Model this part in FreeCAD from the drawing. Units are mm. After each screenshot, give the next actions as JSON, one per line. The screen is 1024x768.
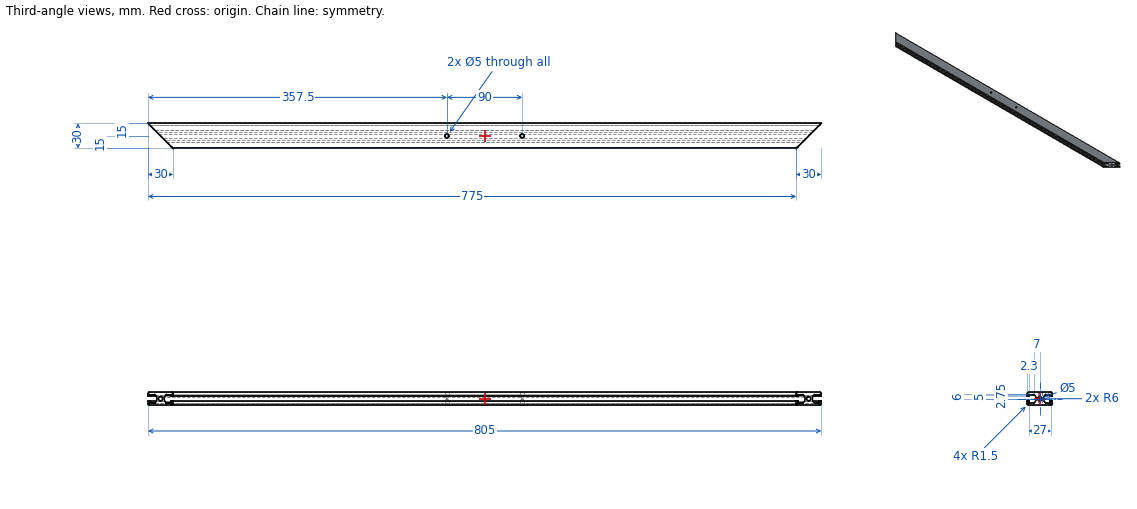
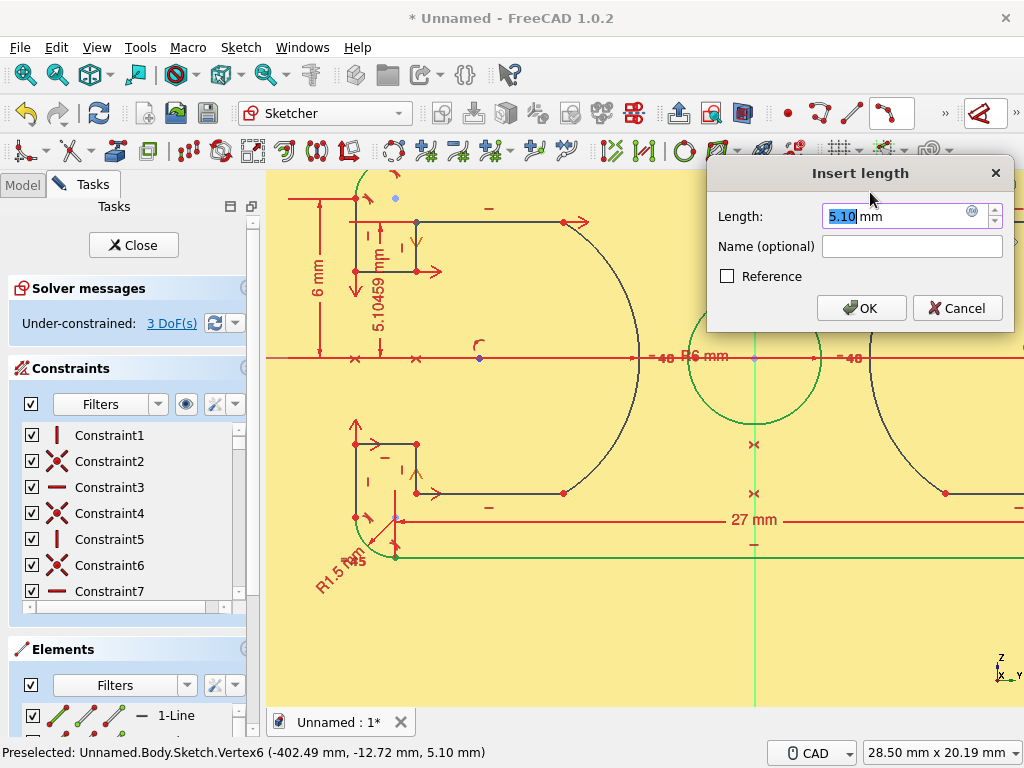
{"action": "type", "text": "5"}
{"action": "key", "text": "Return"}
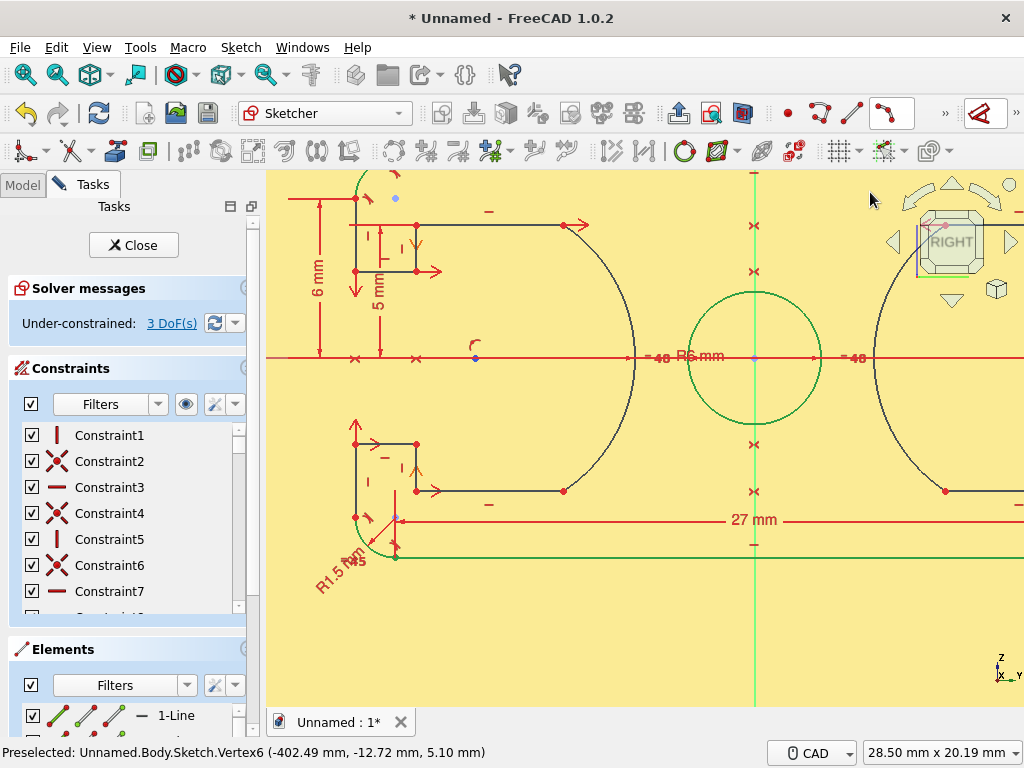
{"action": "left_click", "coordinate": [564, 225]}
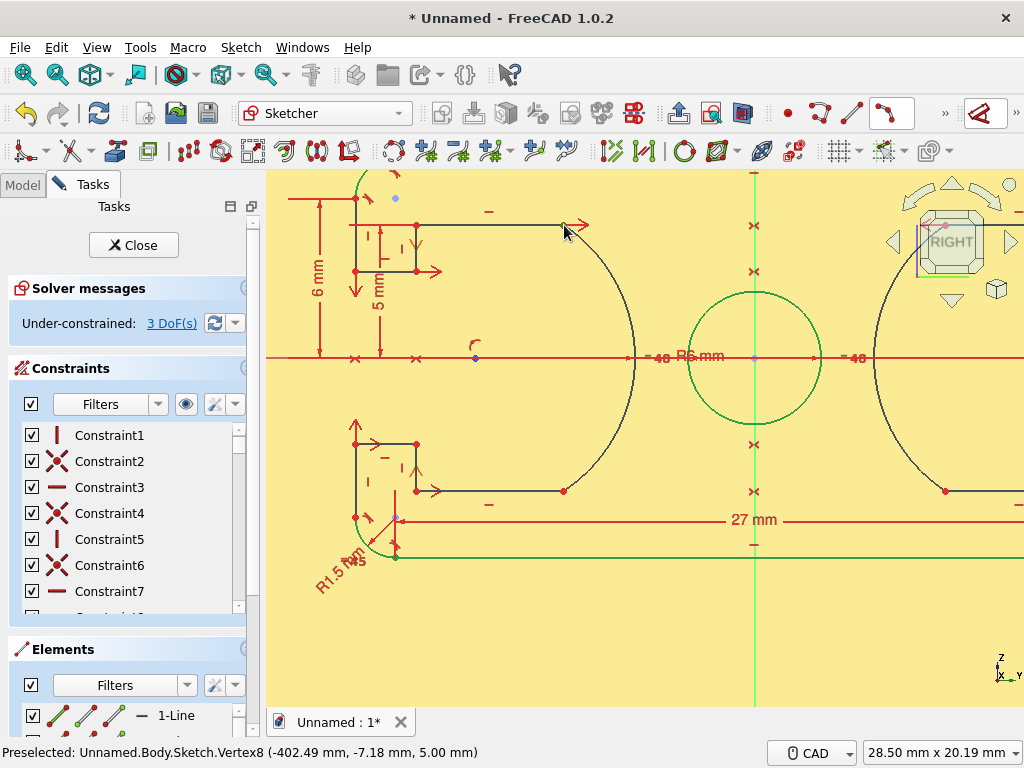
{"action": "left_click", "coordinate": [1002, 114]}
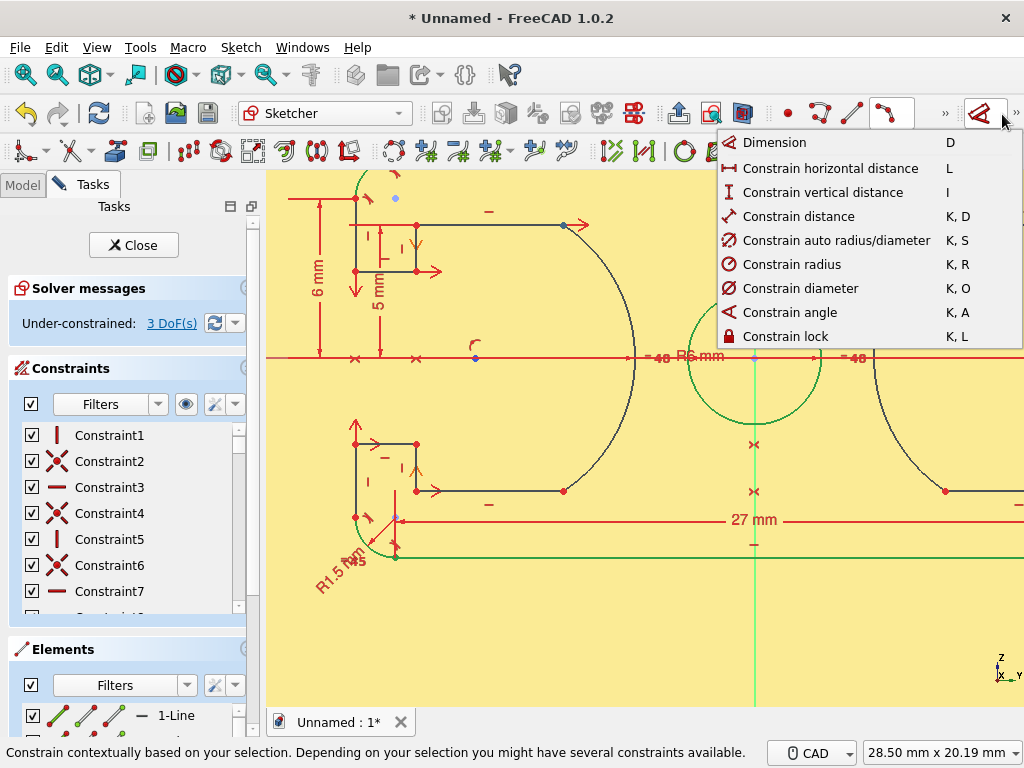
{"action": "left_click", "coordinate": [870, 168]}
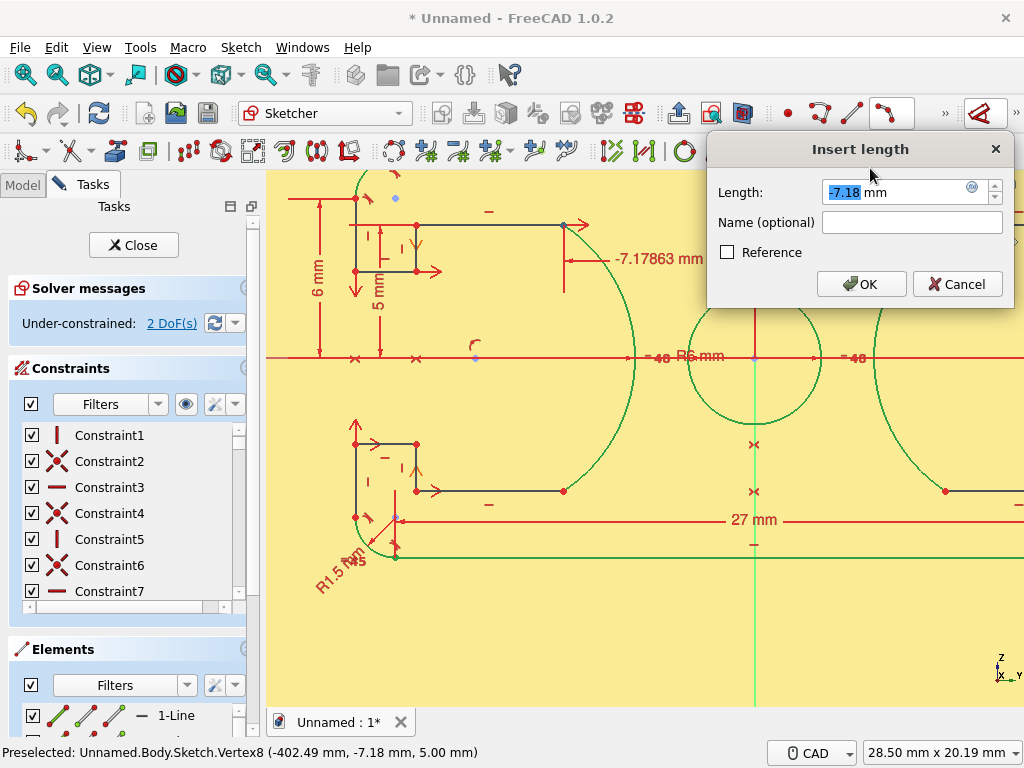
{"action": "type", "text": "-7"}
{"action": "key", "text": "Return"}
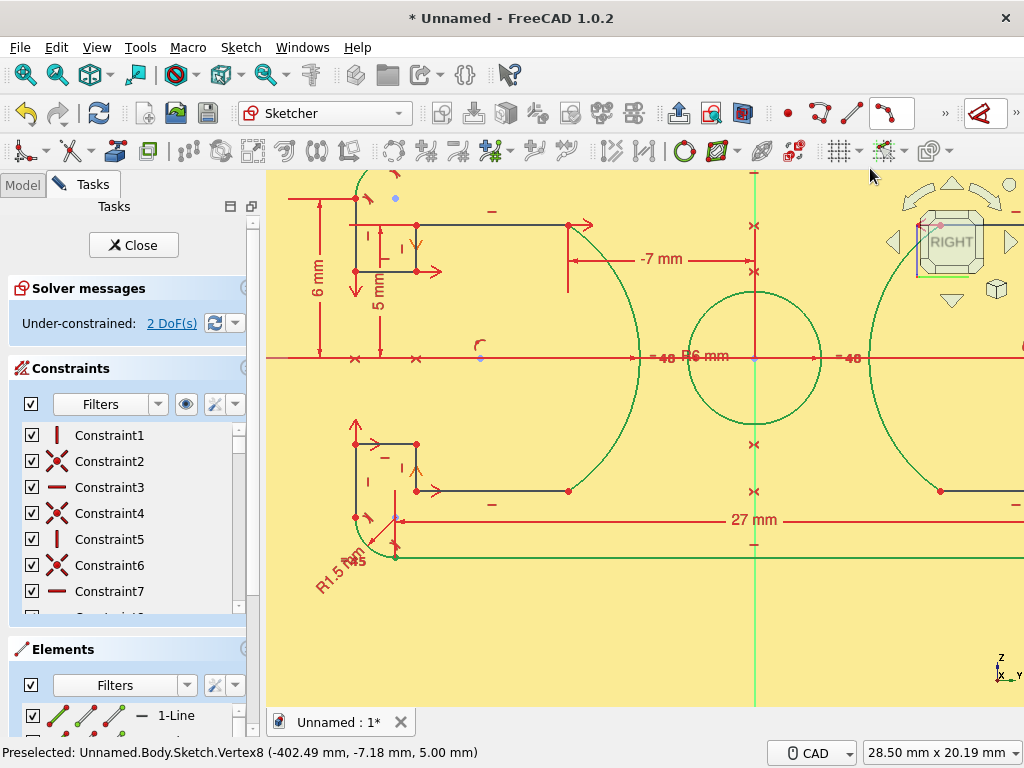
{"action": "left_click", "coordinate": [374, 272]}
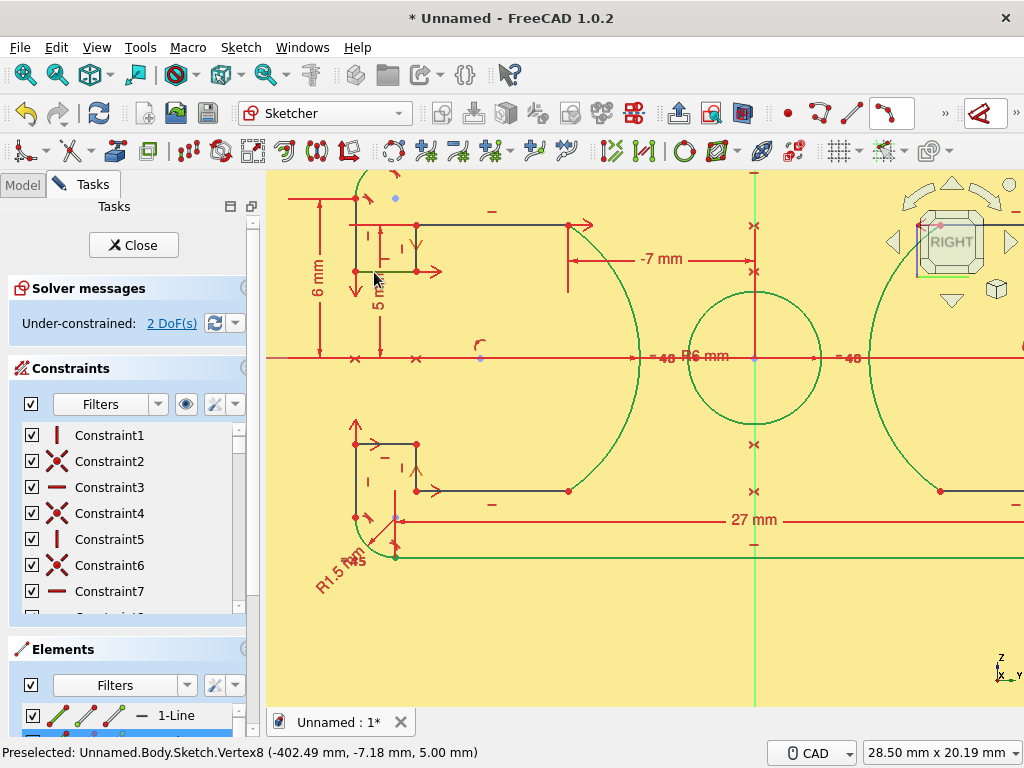
{"action": "left_click", "coordinate": [1002, 114]}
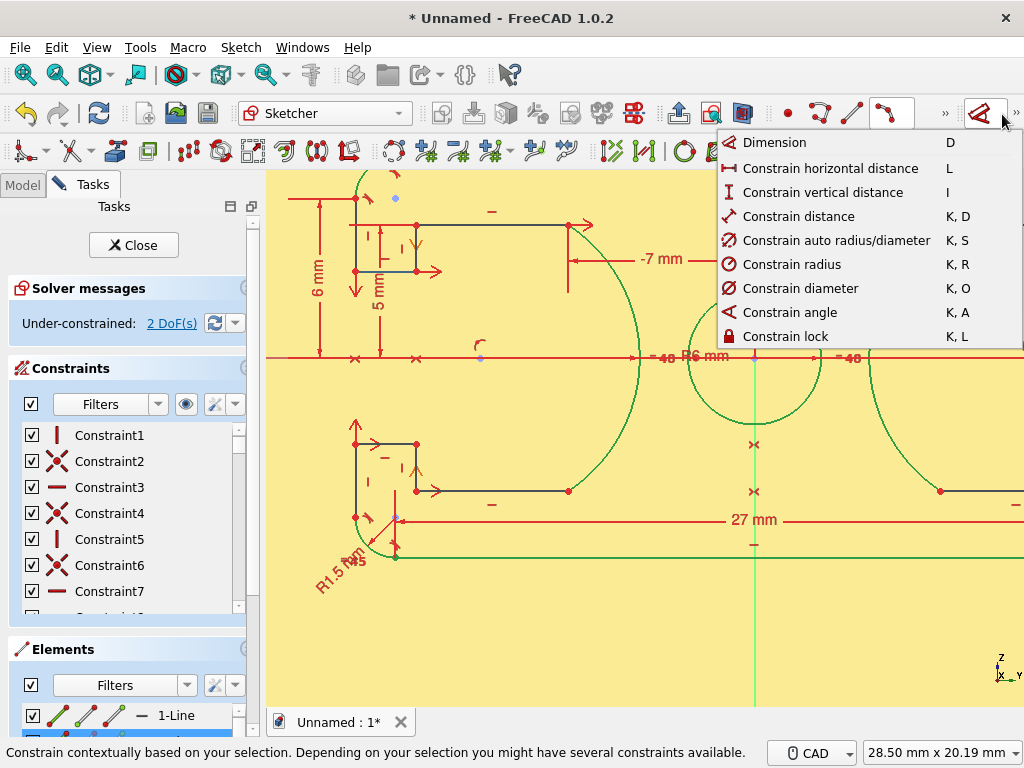
{"action": "left_click", "coordinate": [870, 168]}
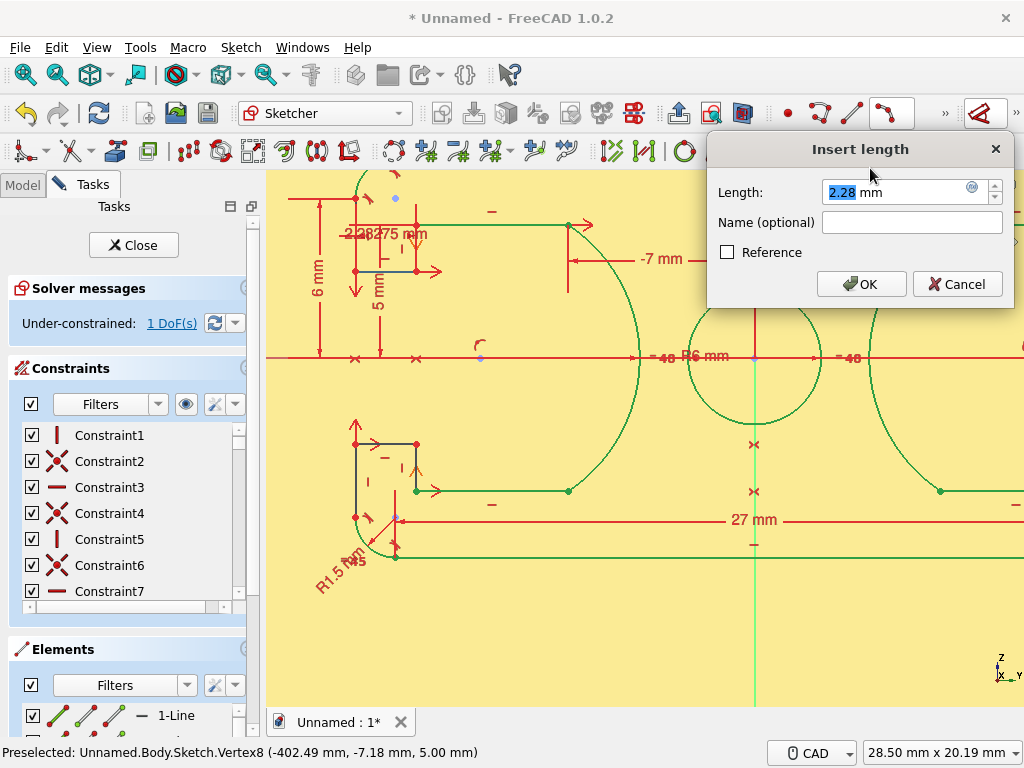
{"action": "type", "text": "2.3"}
{"action": "key", "text": "Return"}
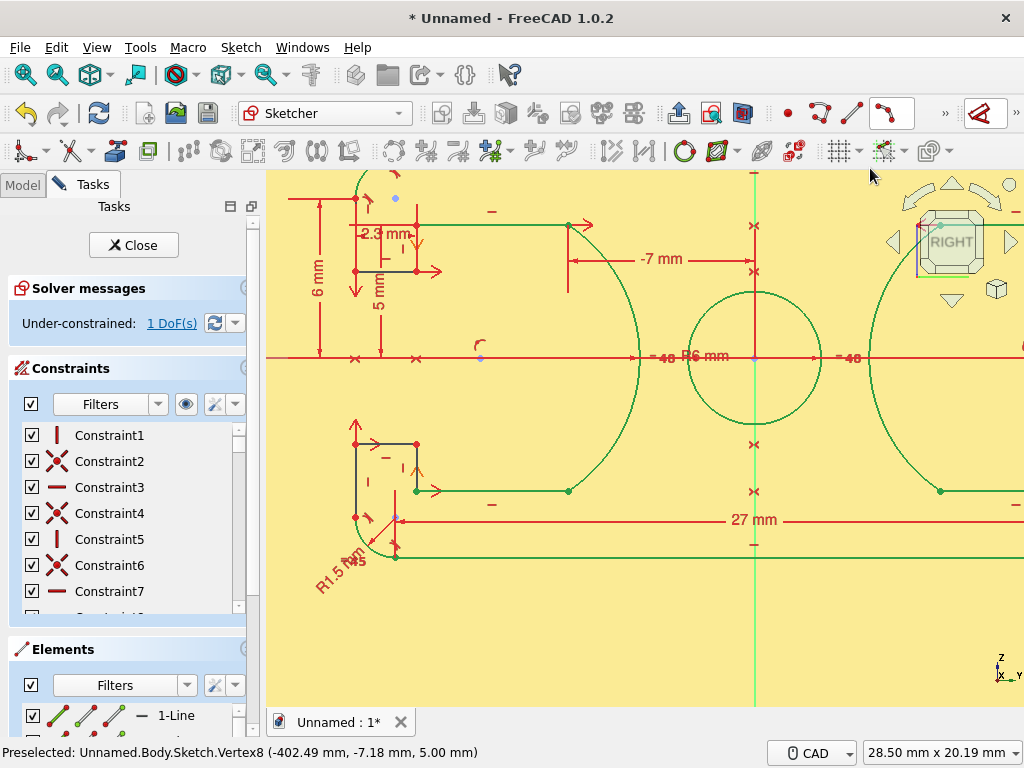
{"action": "left_click", "coordinate": [356, 220]}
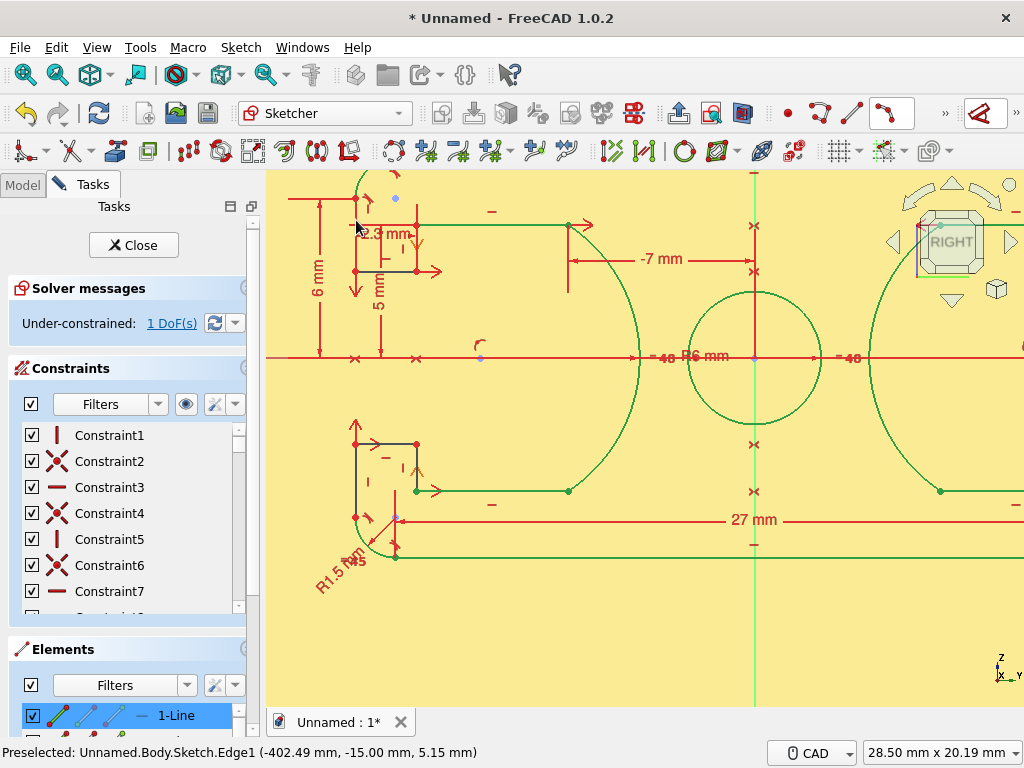
{"action": "key", "text": "i"}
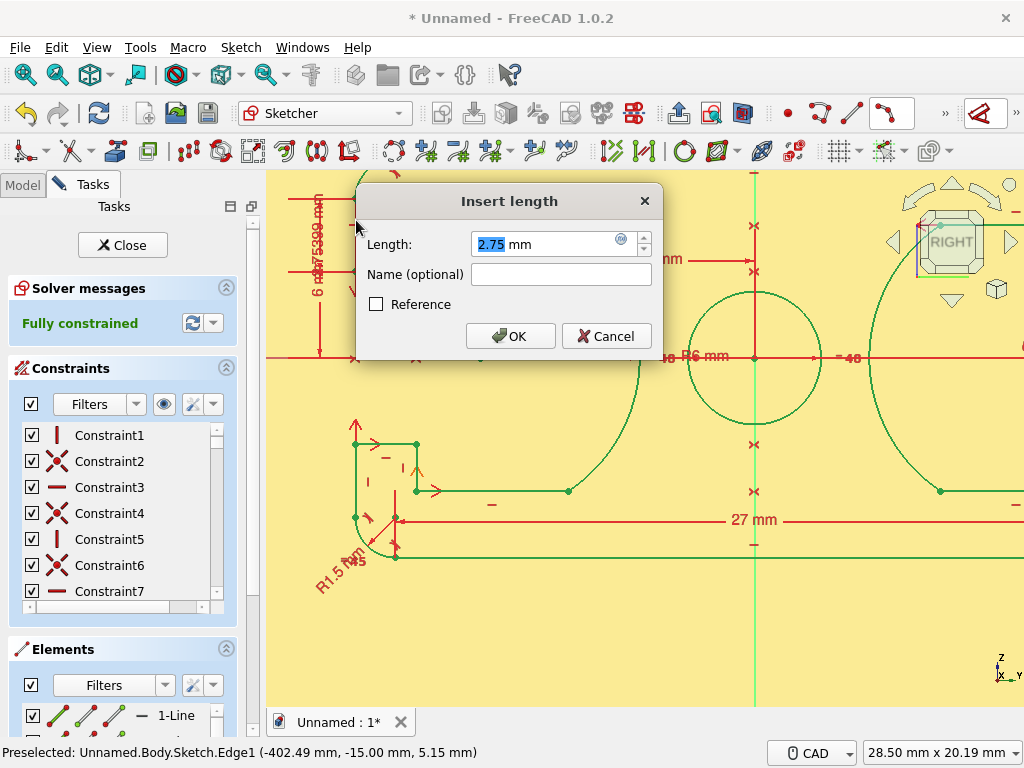
{"action": "type", "text": "2.75"}
{"action": "key", "text": "Return"}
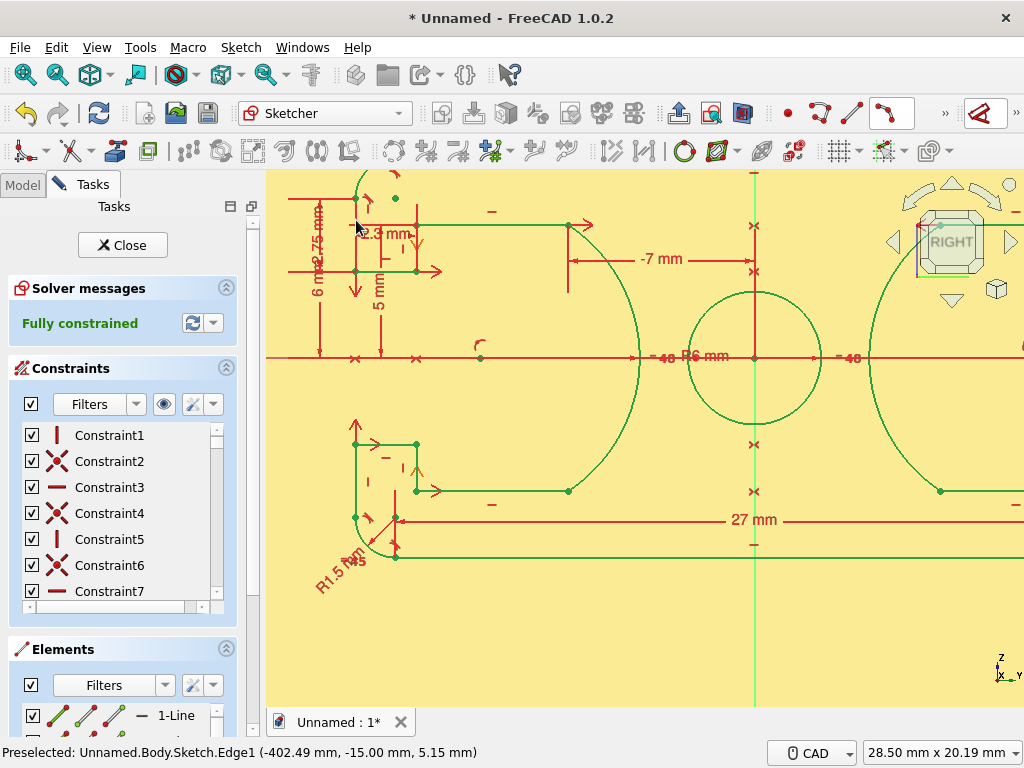
{"action": "left_click", "coordinate": [123, 245]}